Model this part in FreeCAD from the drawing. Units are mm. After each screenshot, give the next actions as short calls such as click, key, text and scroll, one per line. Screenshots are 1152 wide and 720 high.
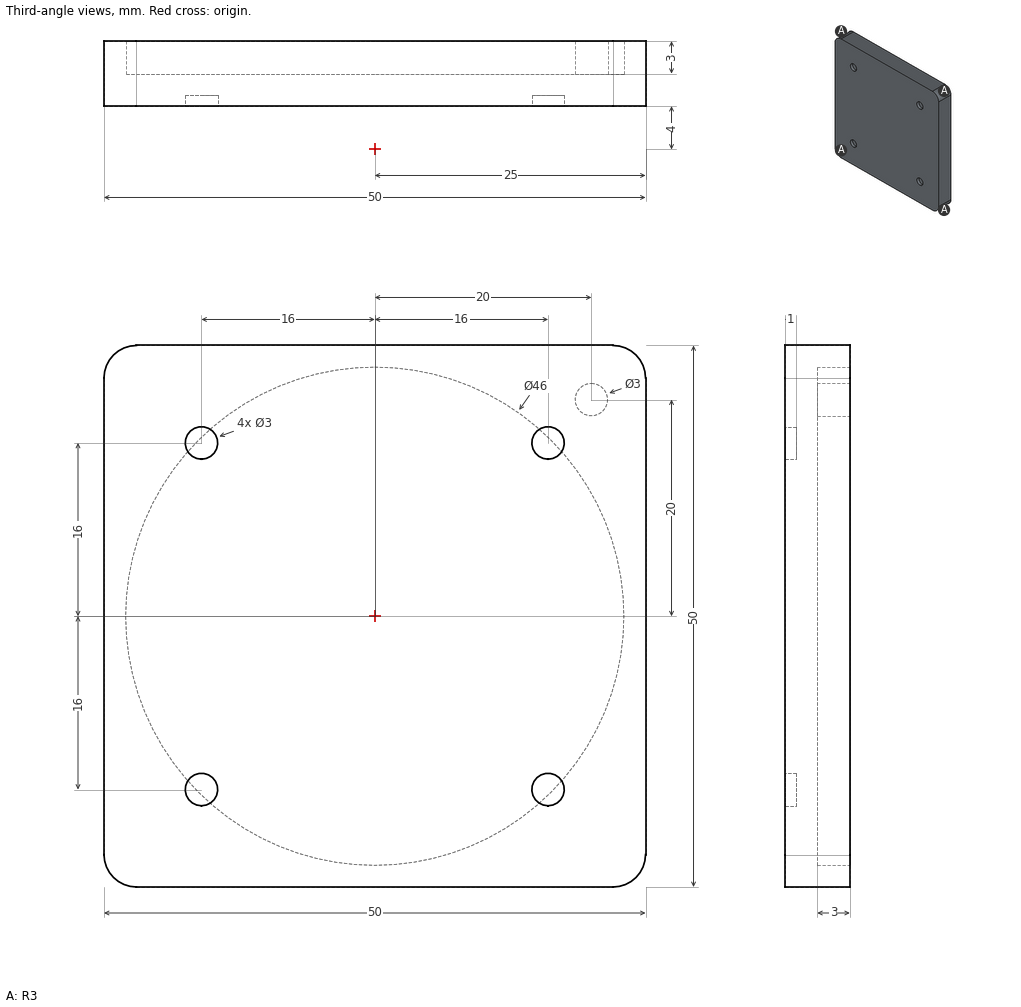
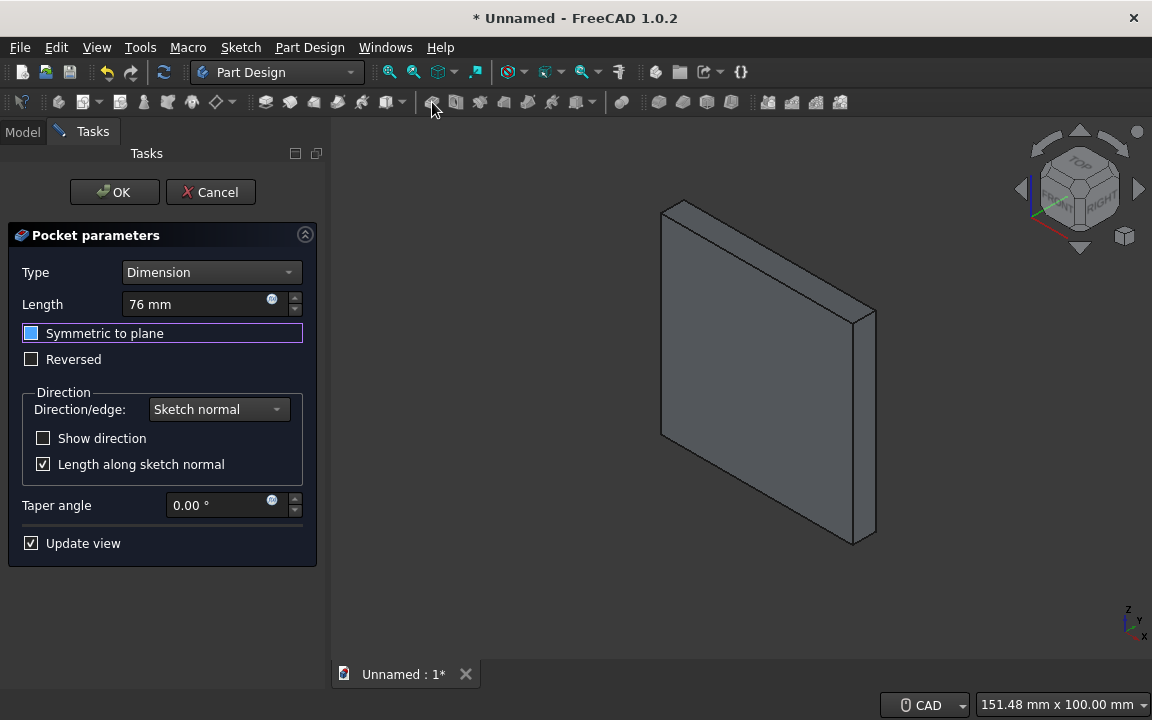
click(115, 192)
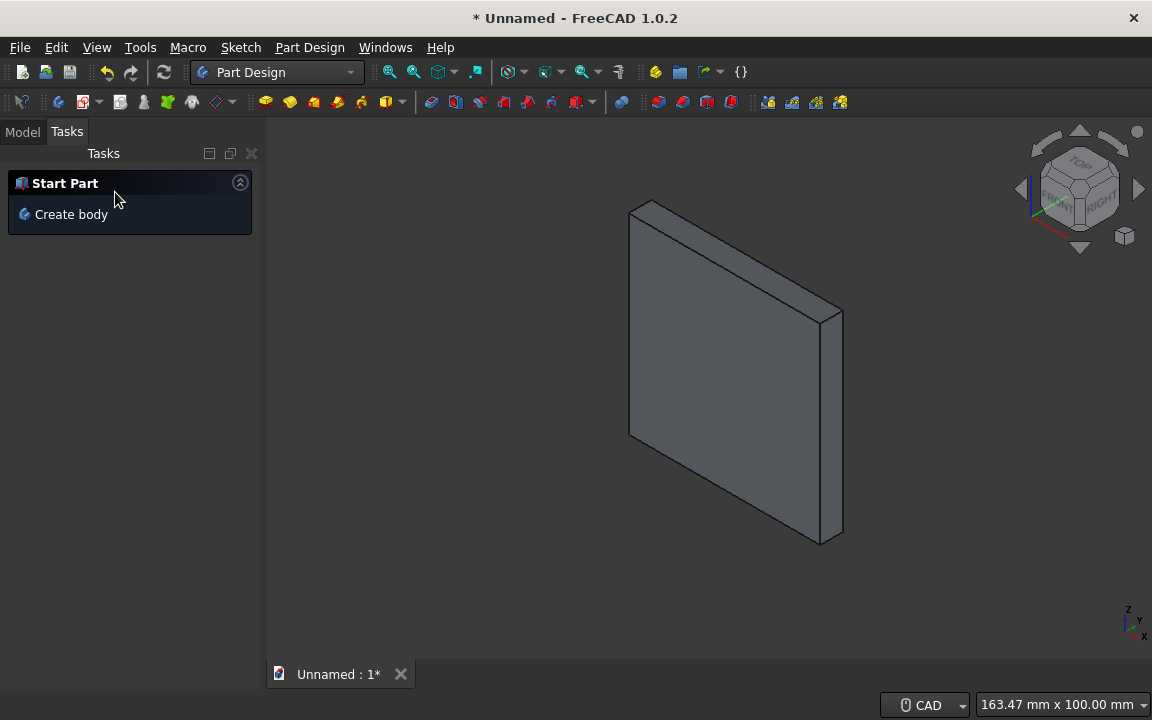
click(832, 316)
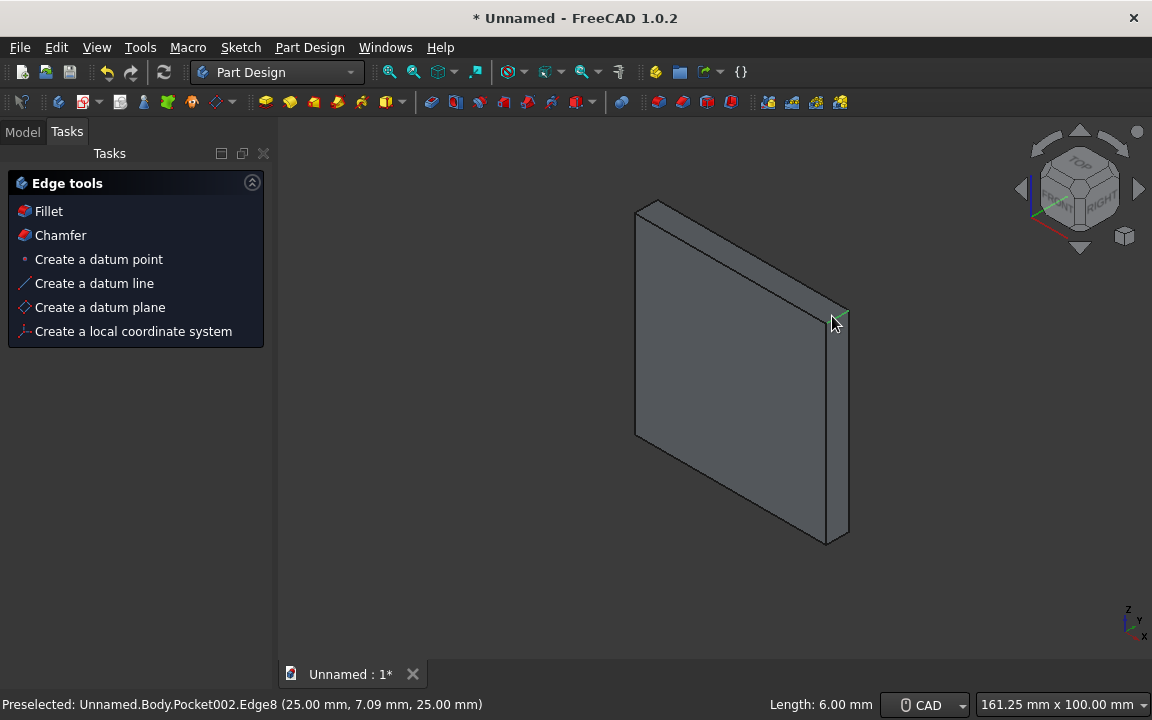
key(2)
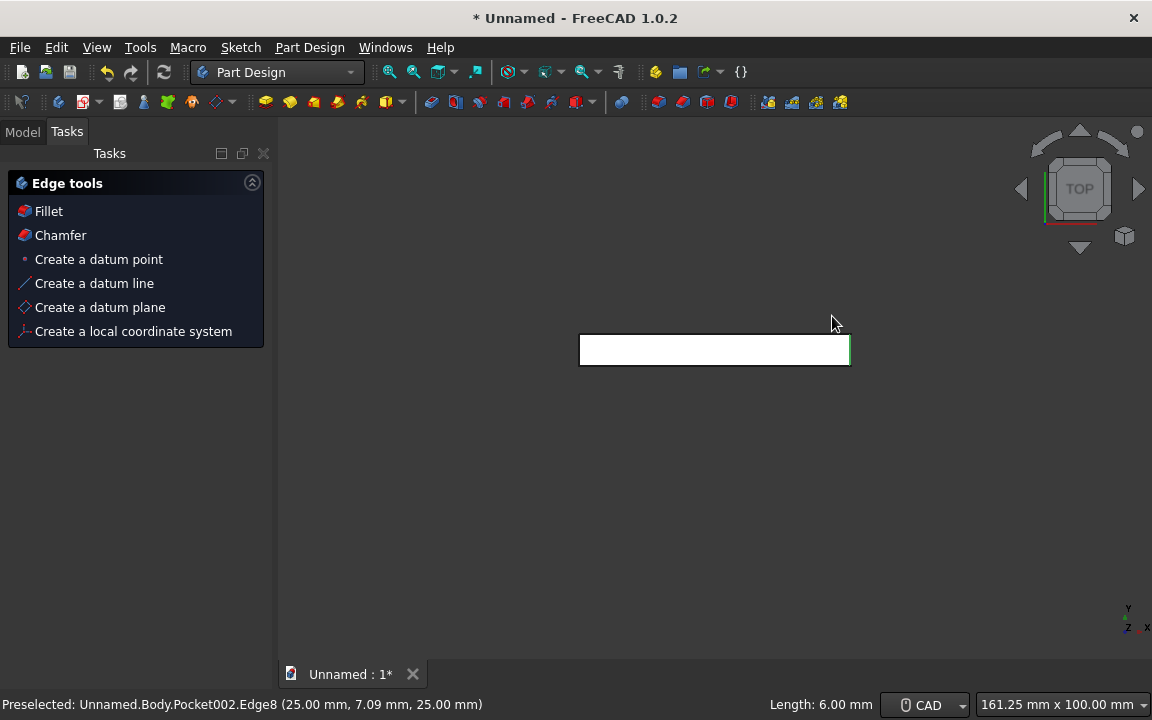
key(v)
key(f)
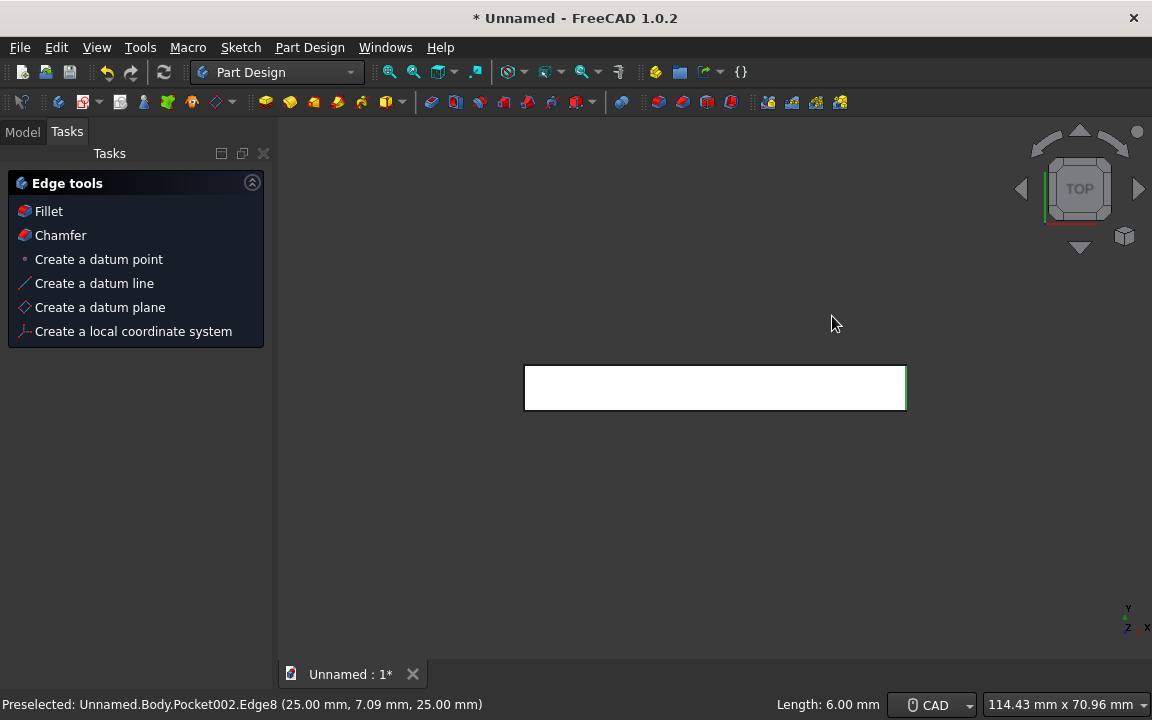
click(524, 387, ctrl)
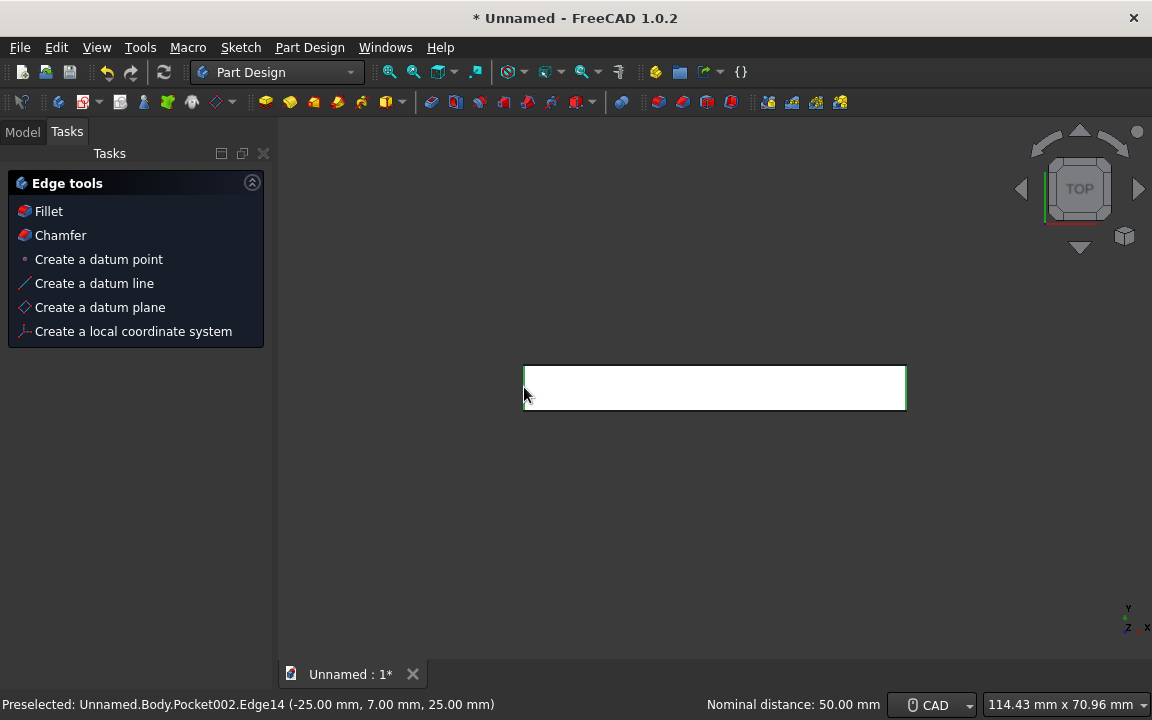
key(0)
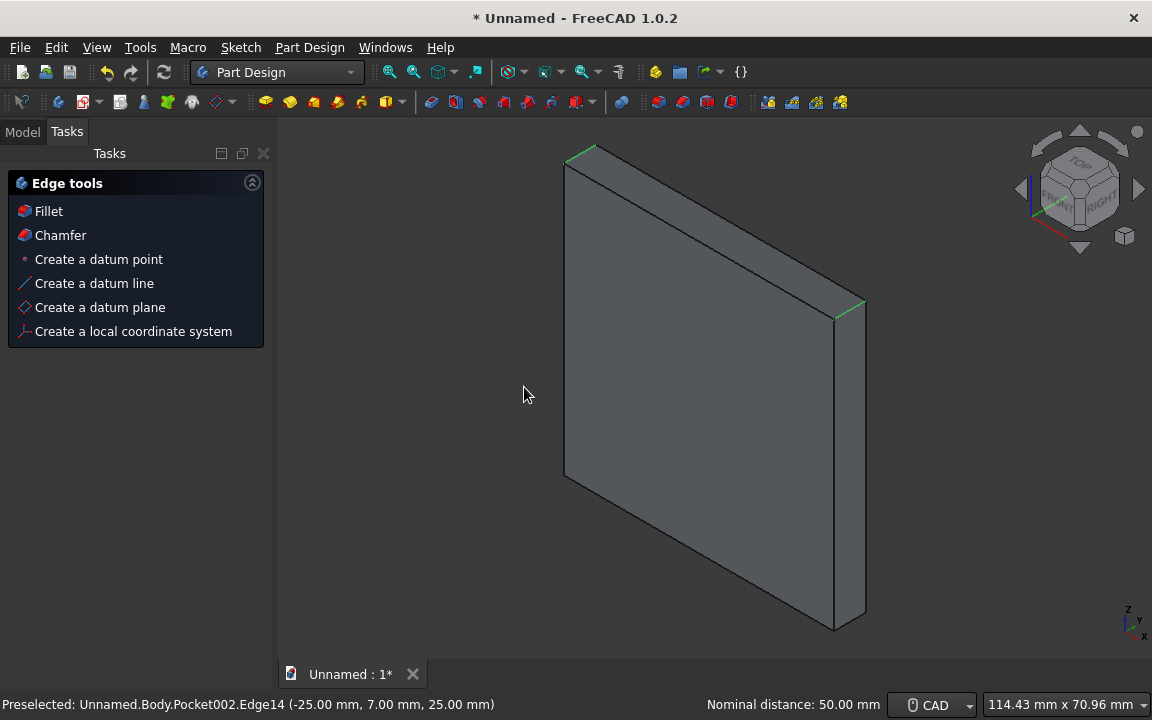
key(1)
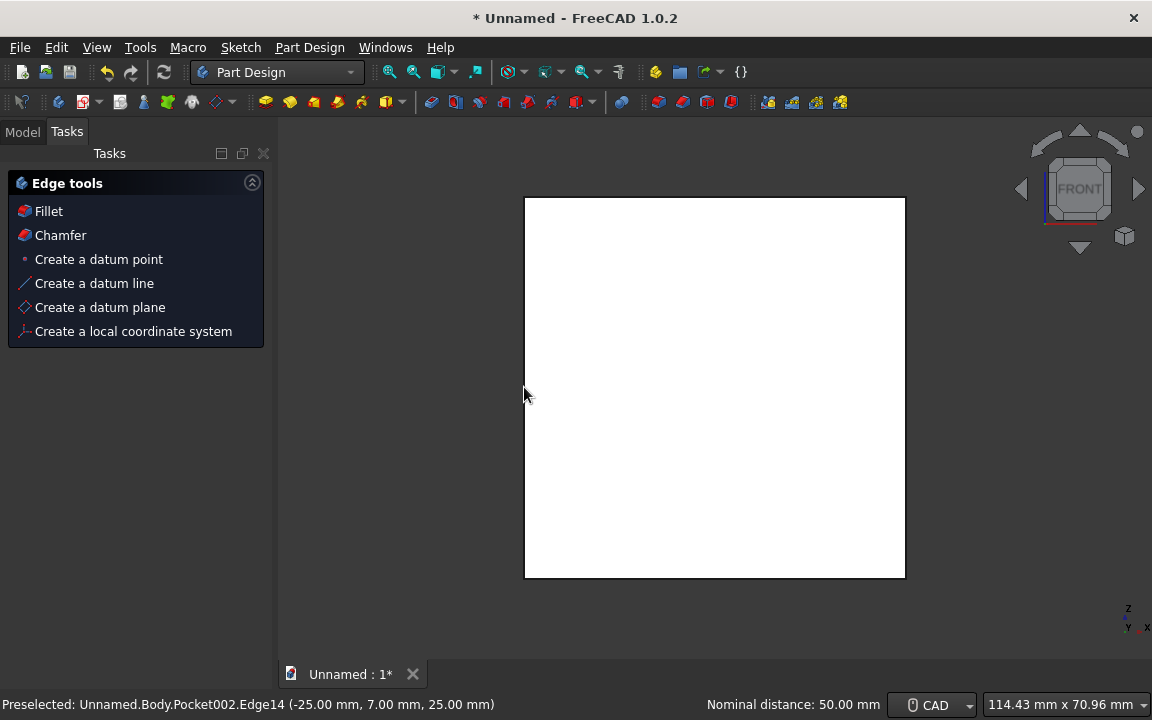
key(3)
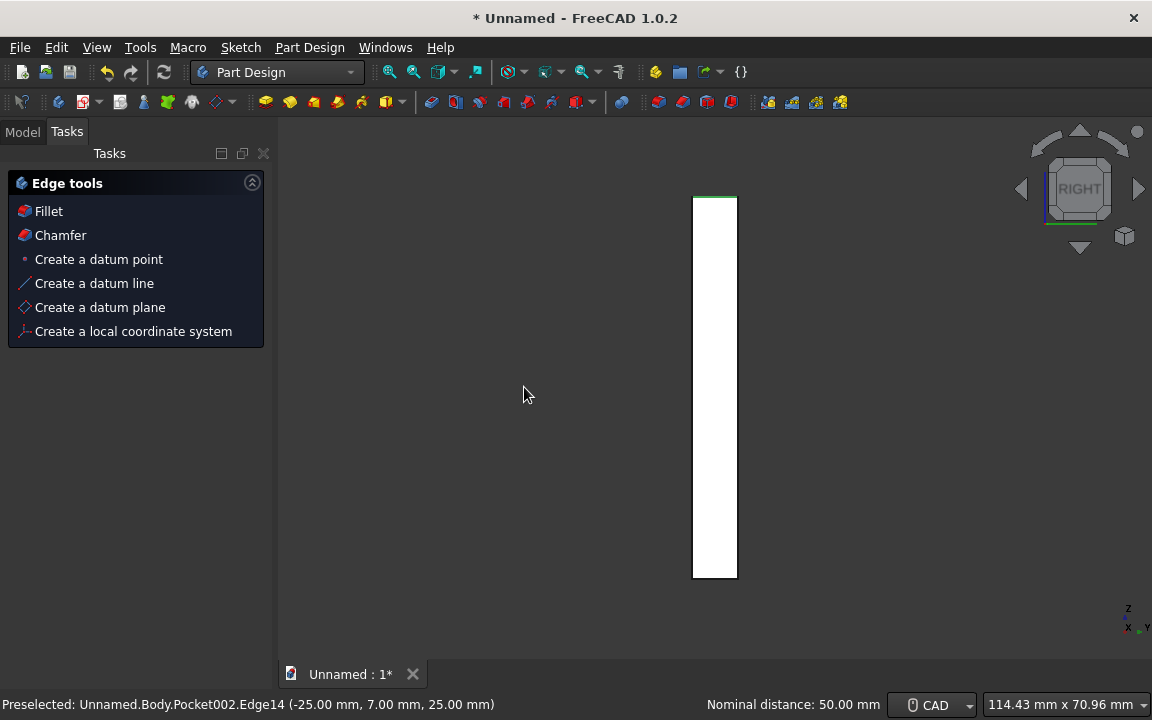
click(715, 578, ctrl)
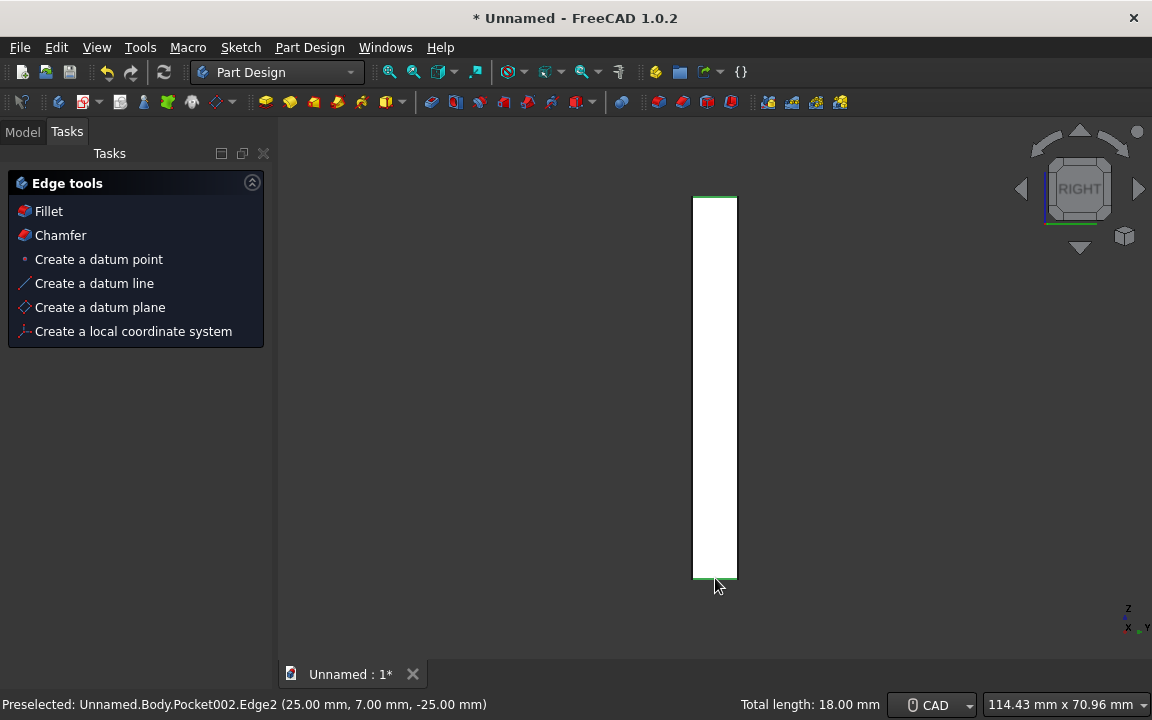
key(5)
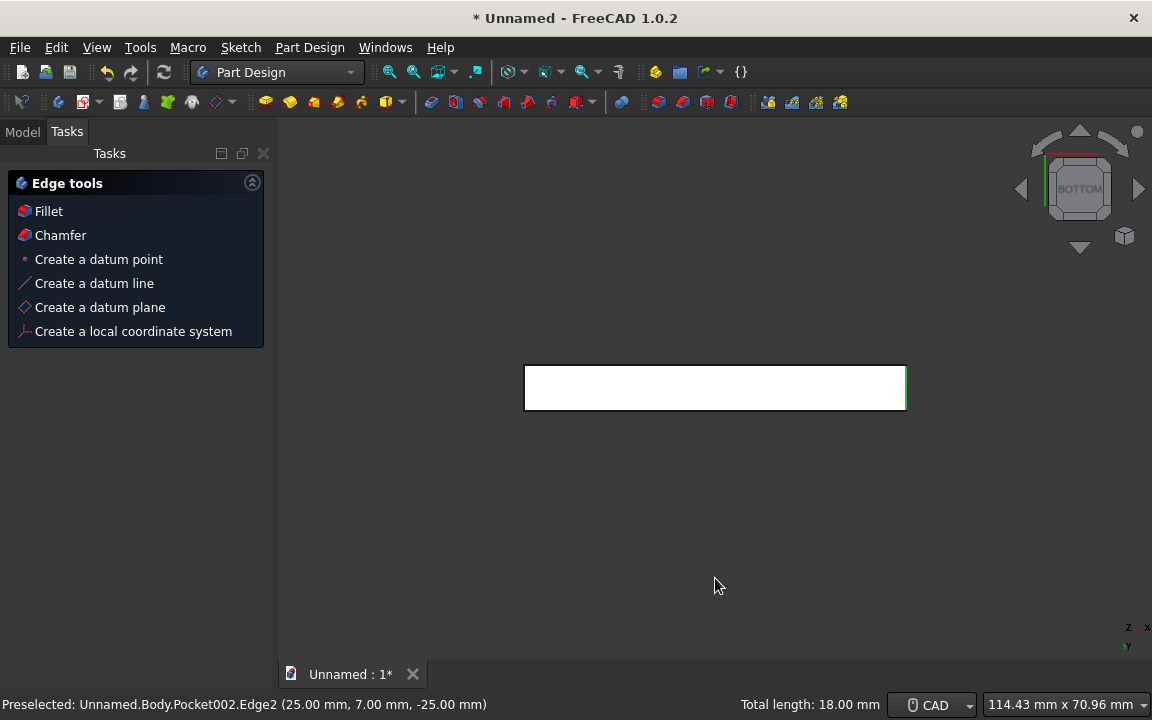
click(390, 72)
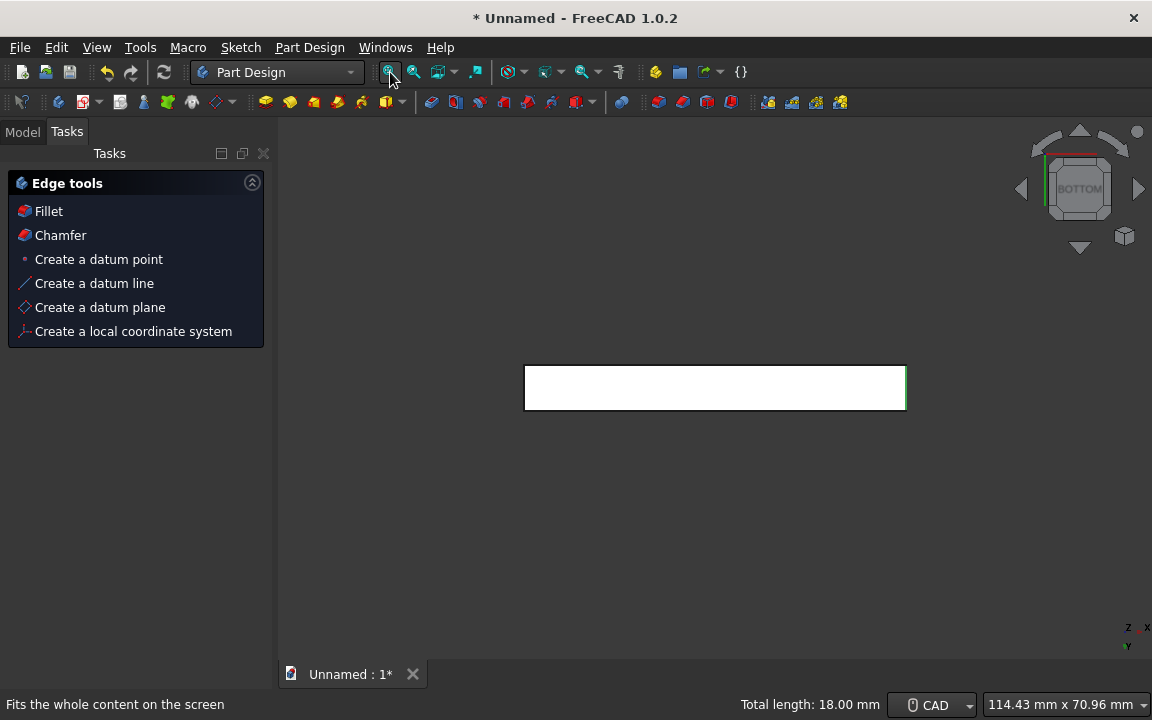
click(524, 387, ctrl)